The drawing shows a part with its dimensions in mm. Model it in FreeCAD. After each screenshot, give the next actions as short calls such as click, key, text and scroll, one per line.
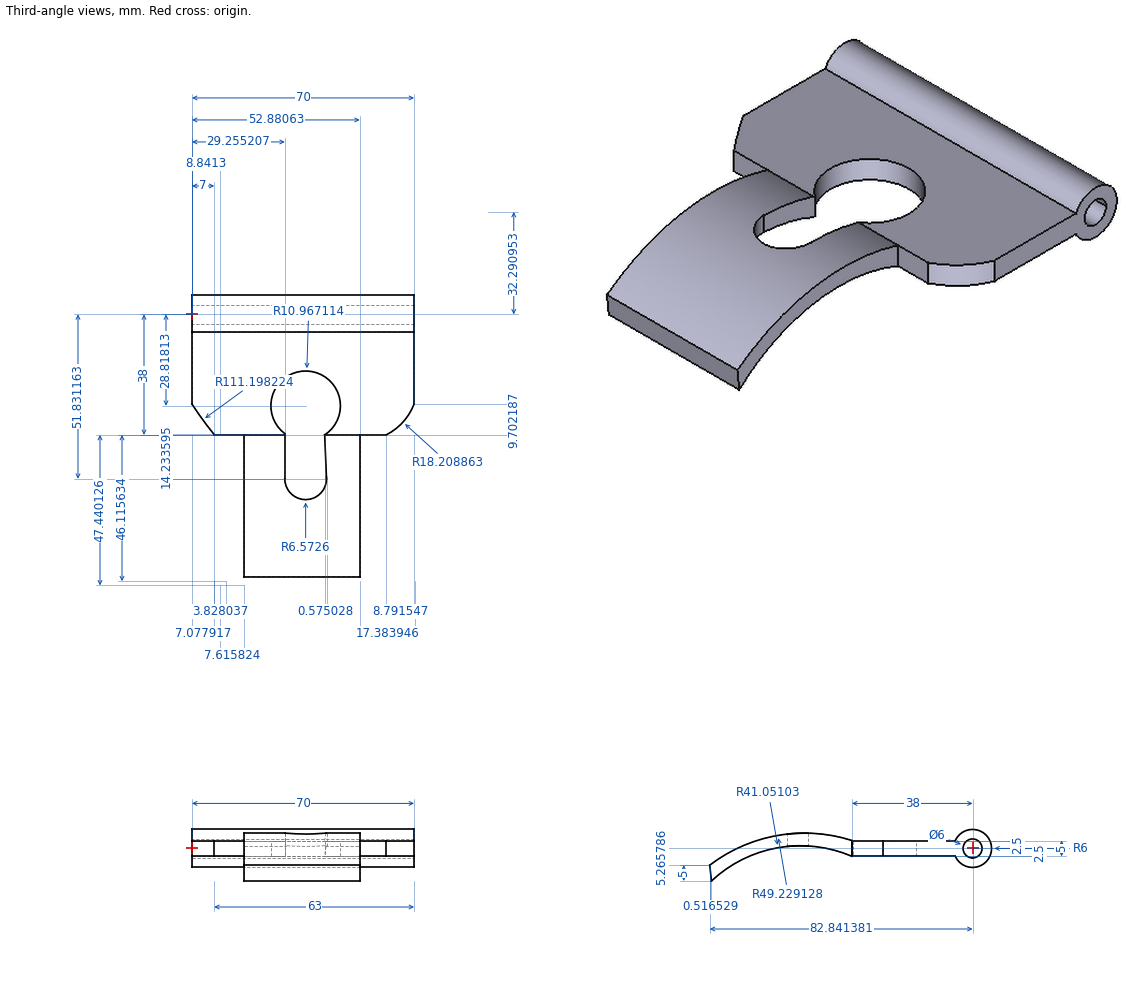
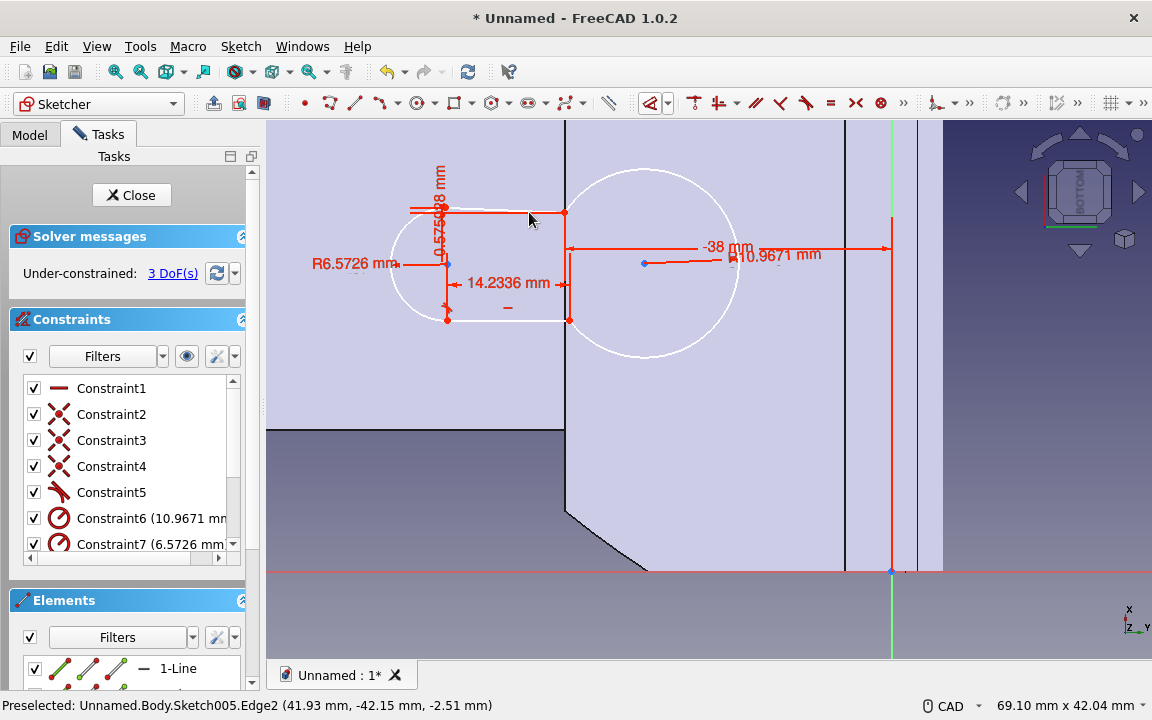
click(644, 263)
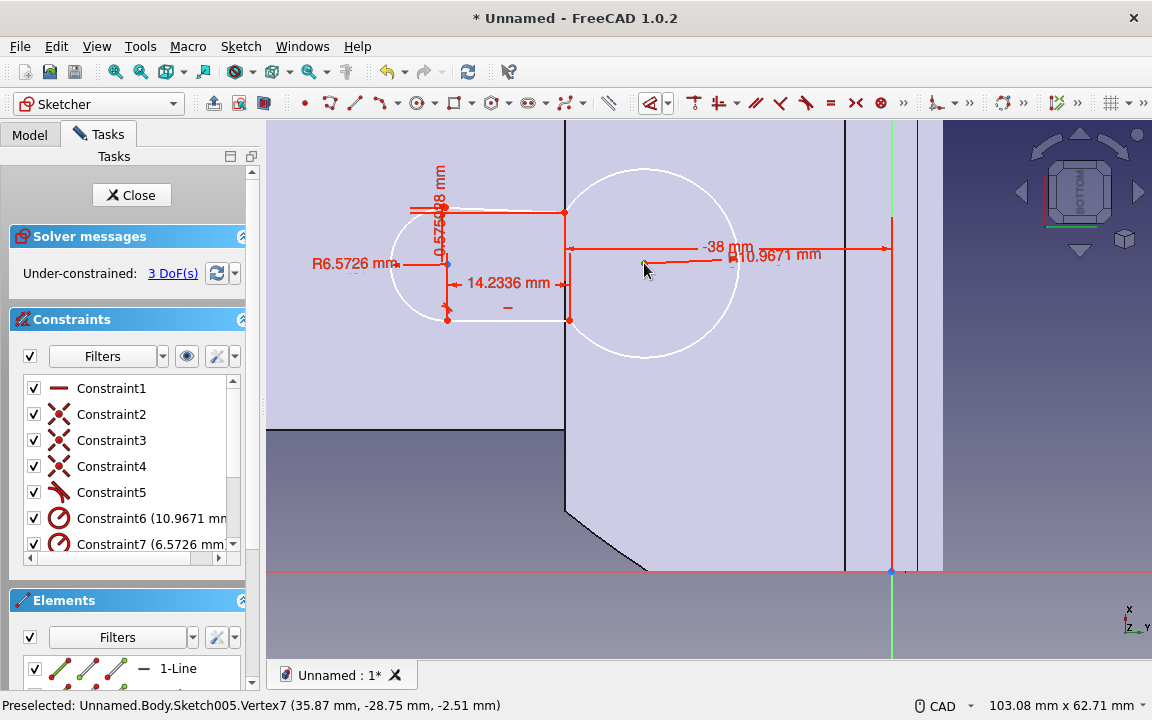
key(l)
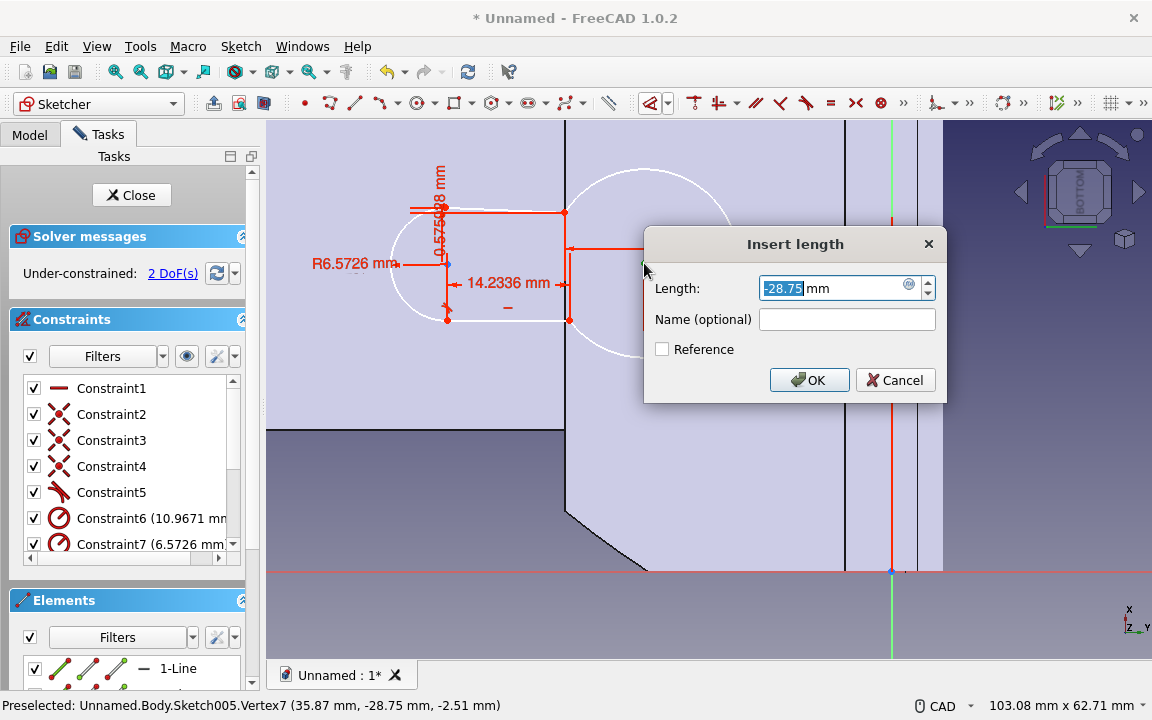
text(-28.81813)
key(Return)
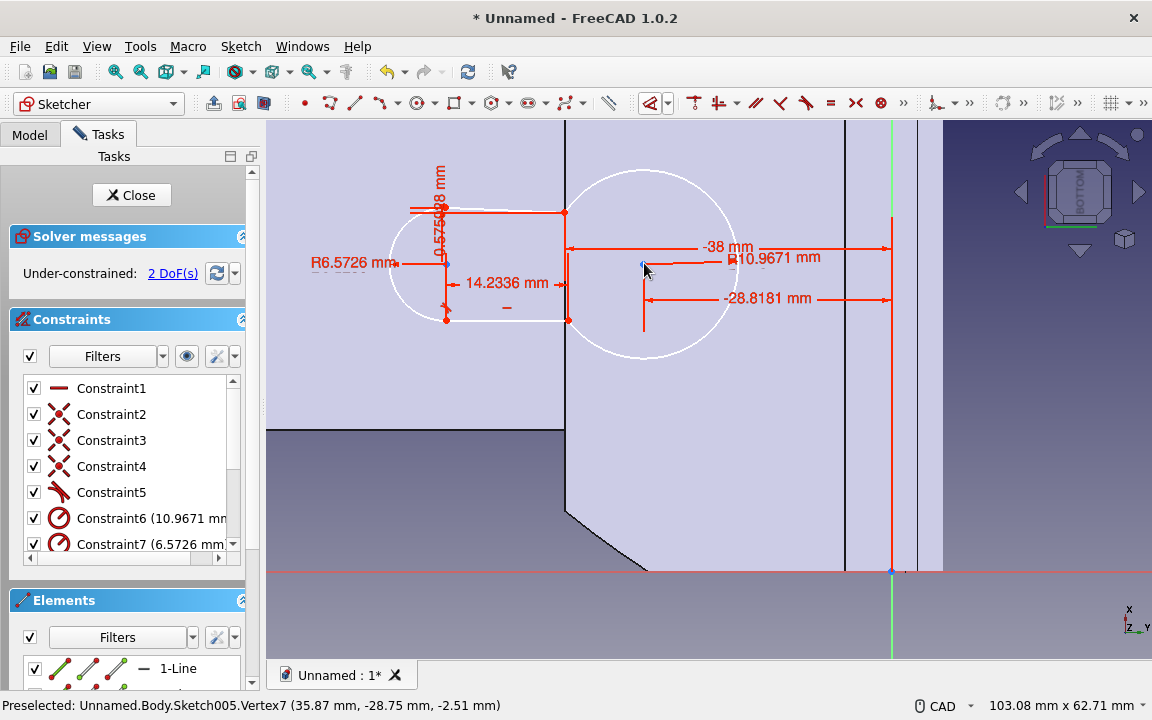
click(446, 321)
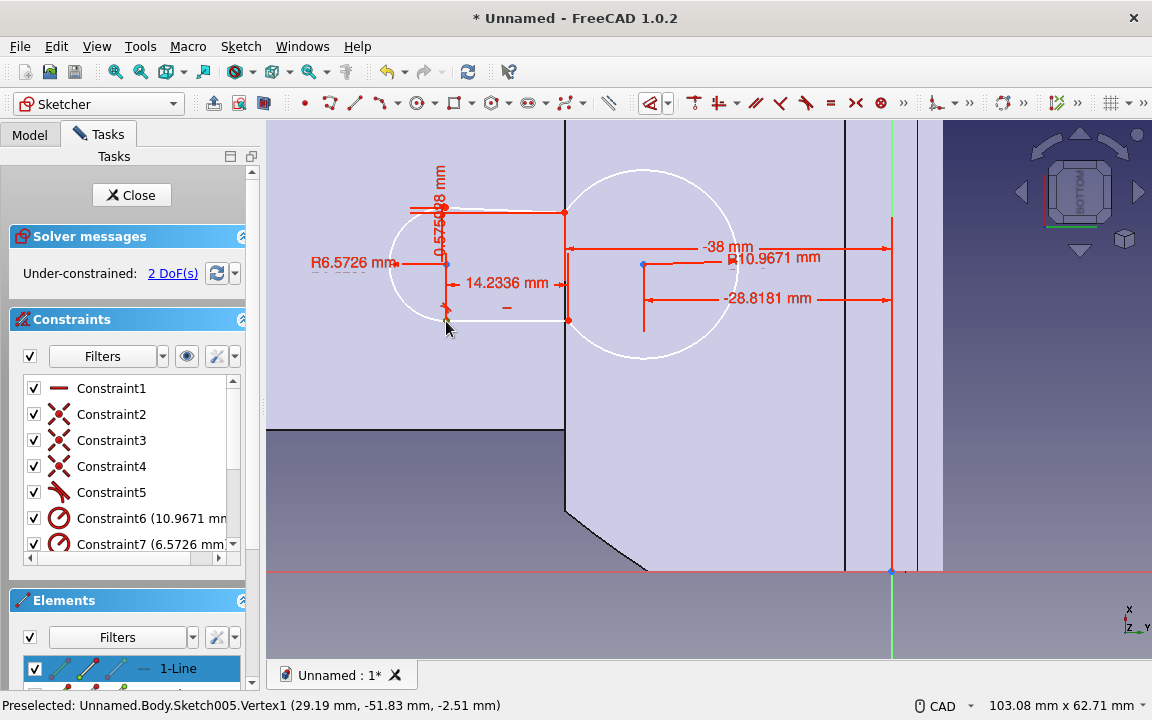
key(i)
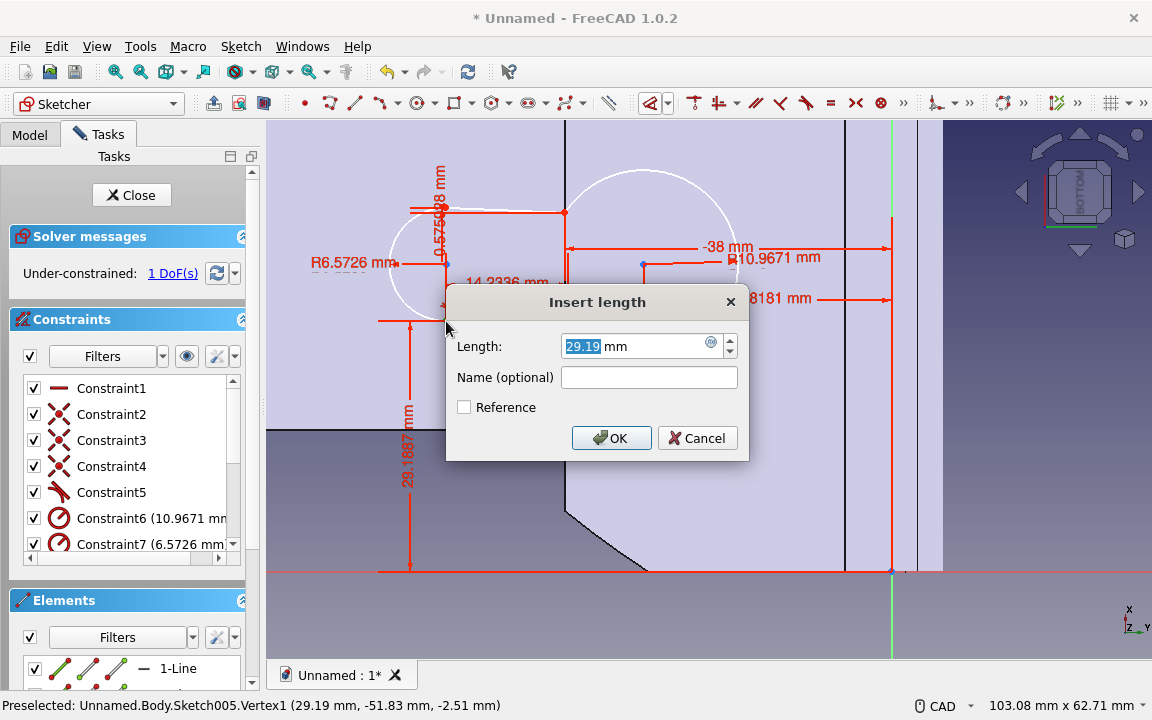
text(29.255207)
key(Return)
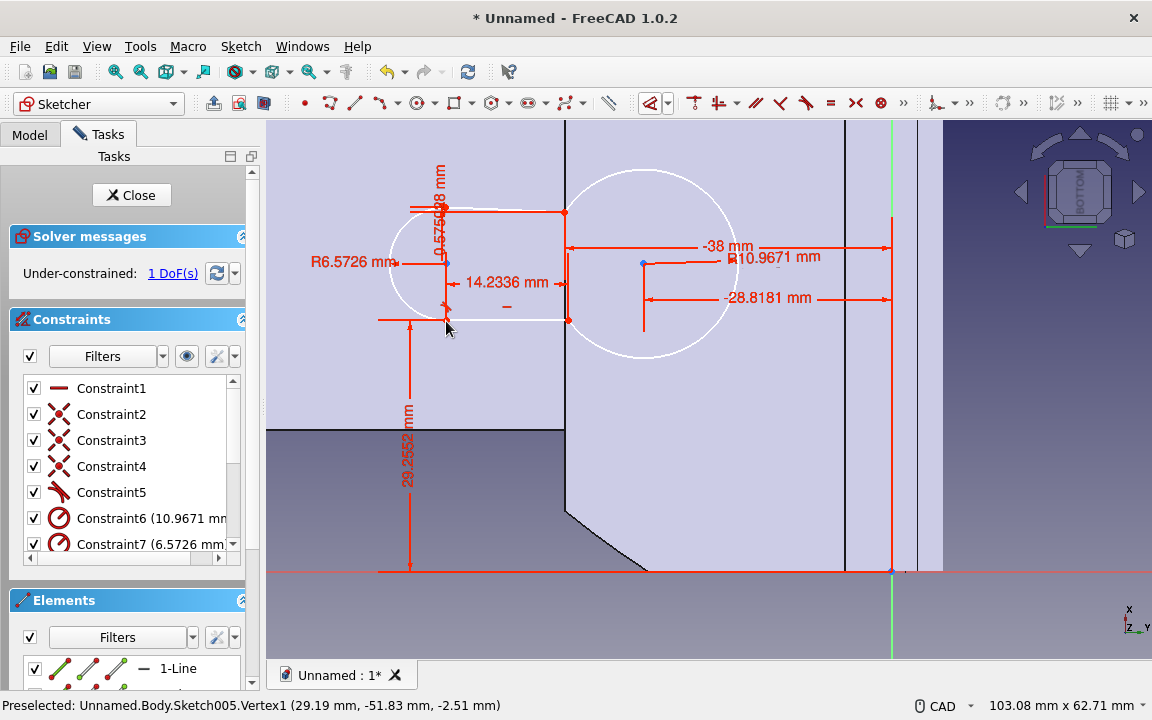
click(446, 207)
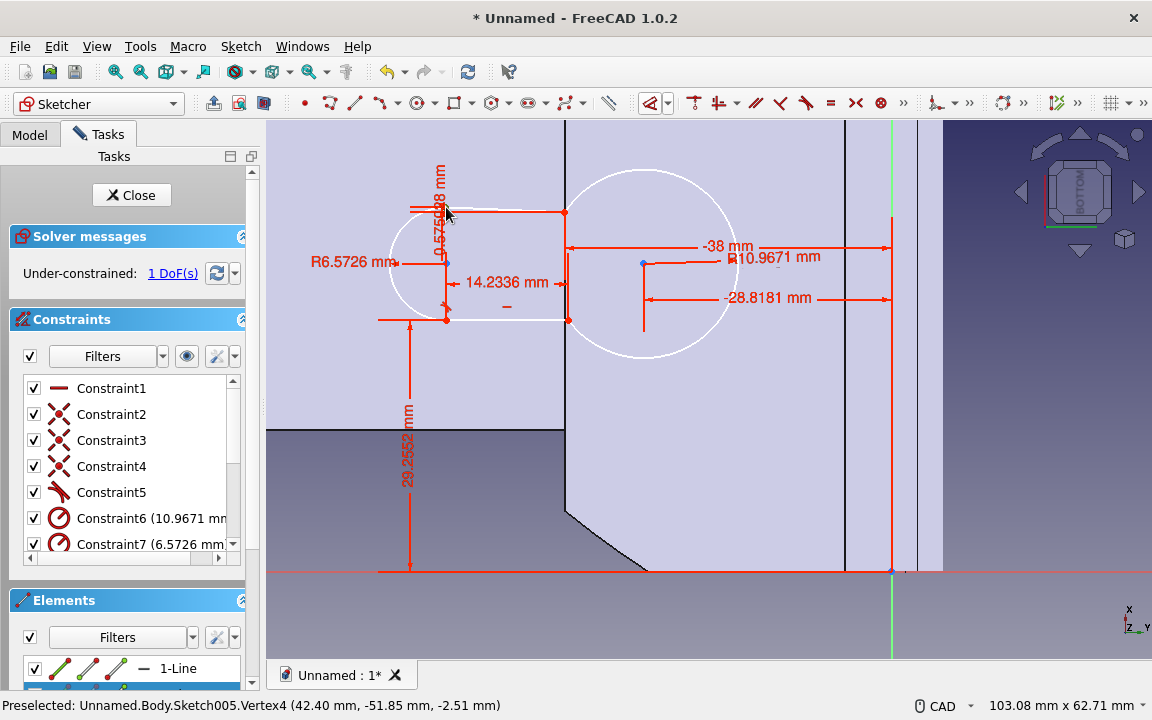
key(l)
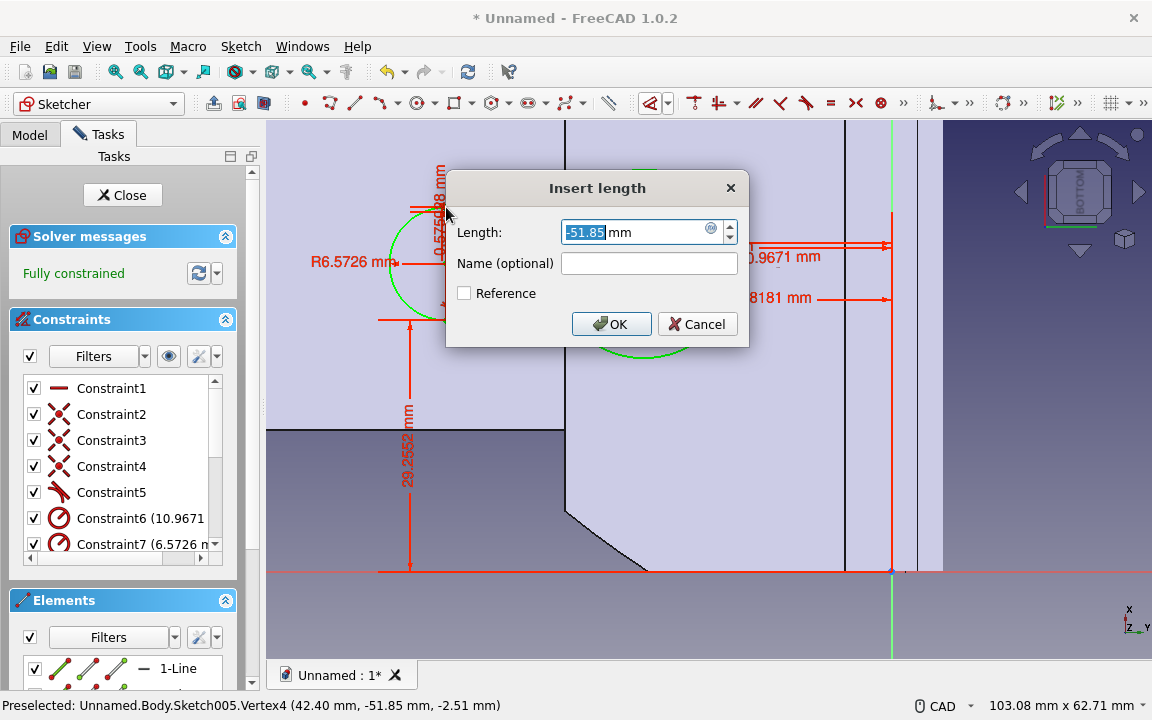
text(-51.831163)
key(Return)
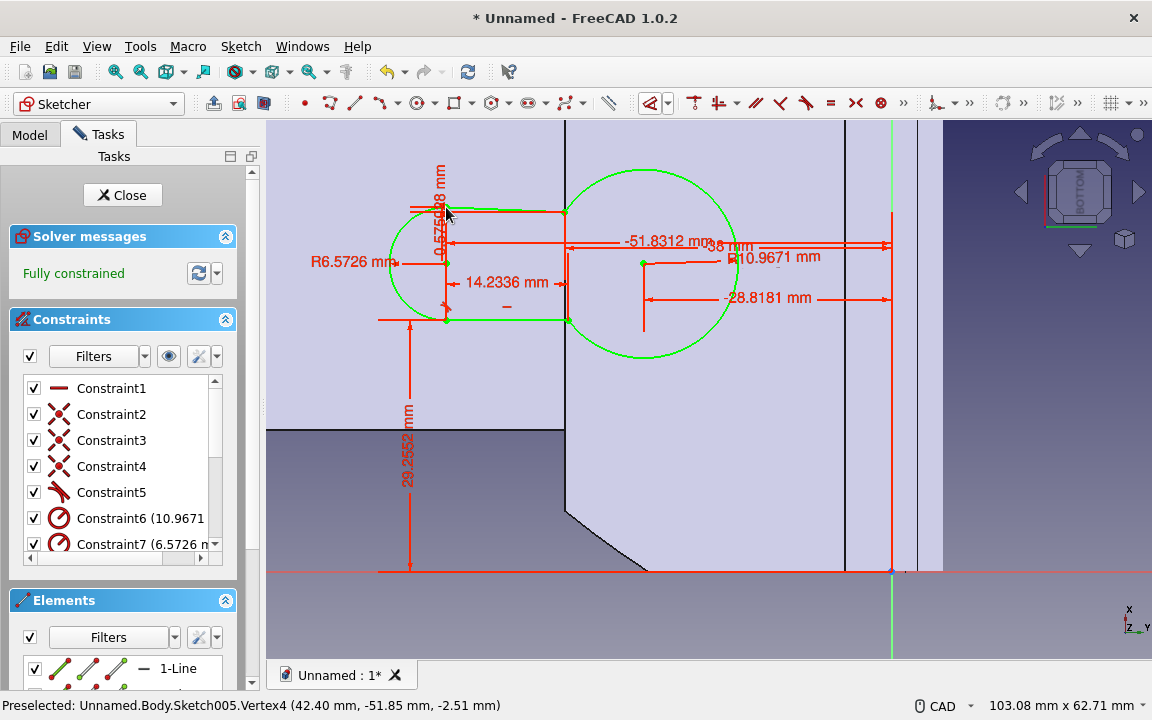
click(123, 195)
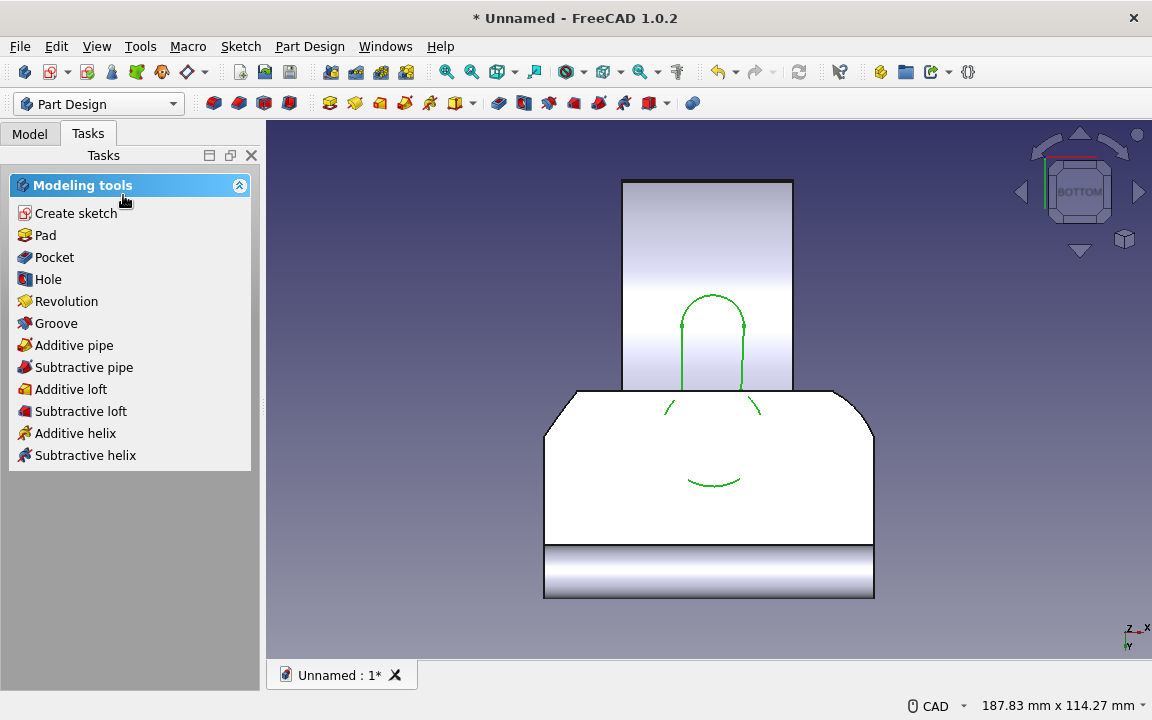
click(499, 104)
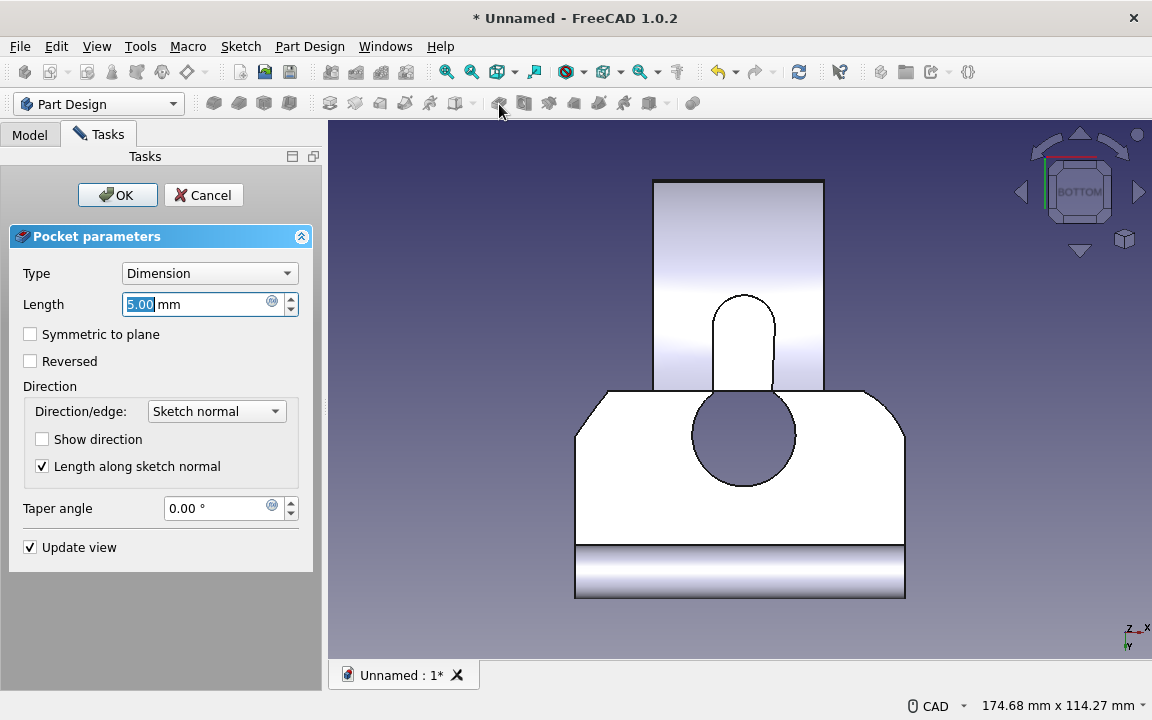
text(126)
key(Tab)